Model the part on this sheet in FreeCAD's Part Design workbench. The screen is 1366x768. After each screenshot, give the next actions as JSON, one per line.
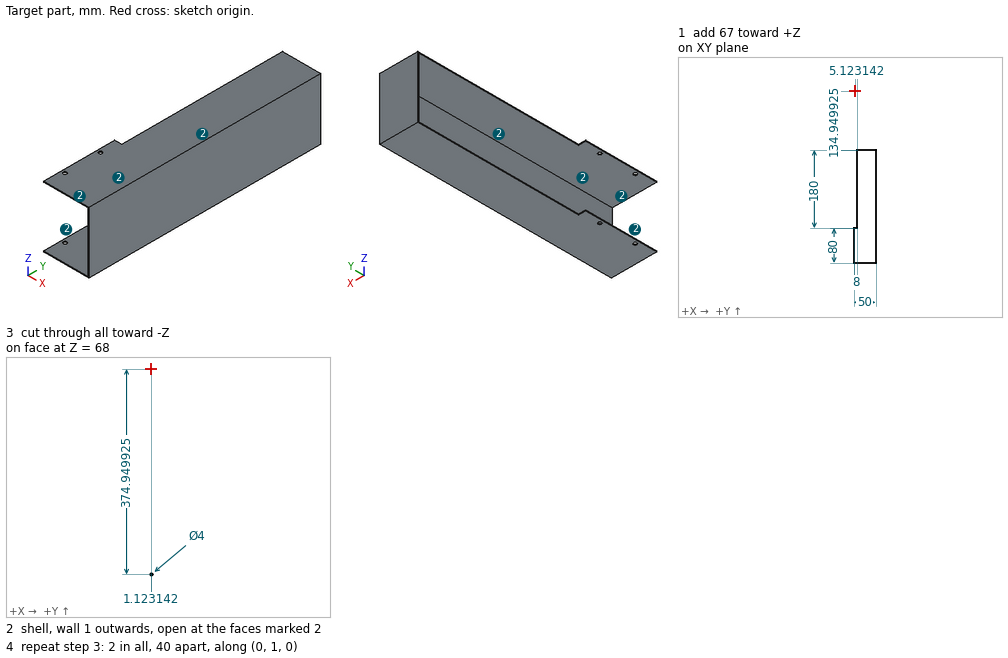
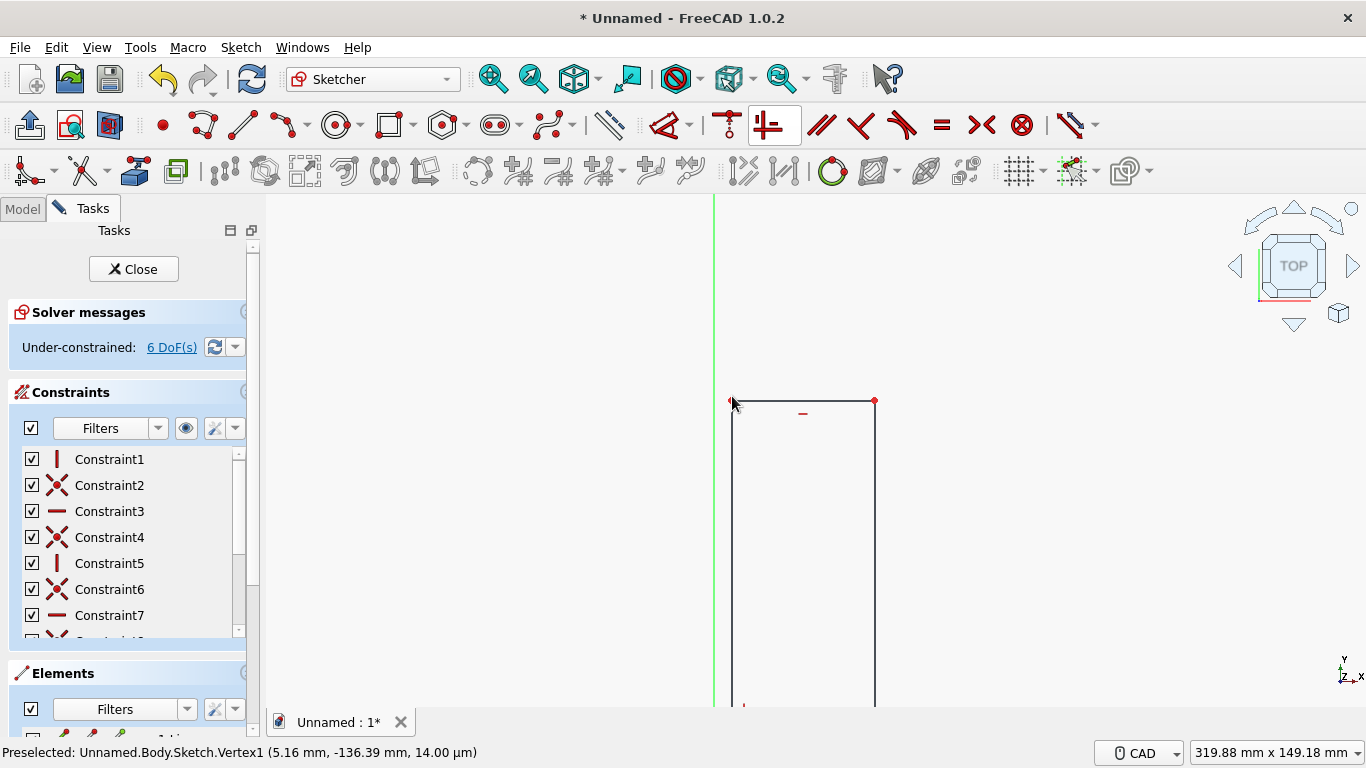
{"action": "left_click", "coordinate": [664, 126]}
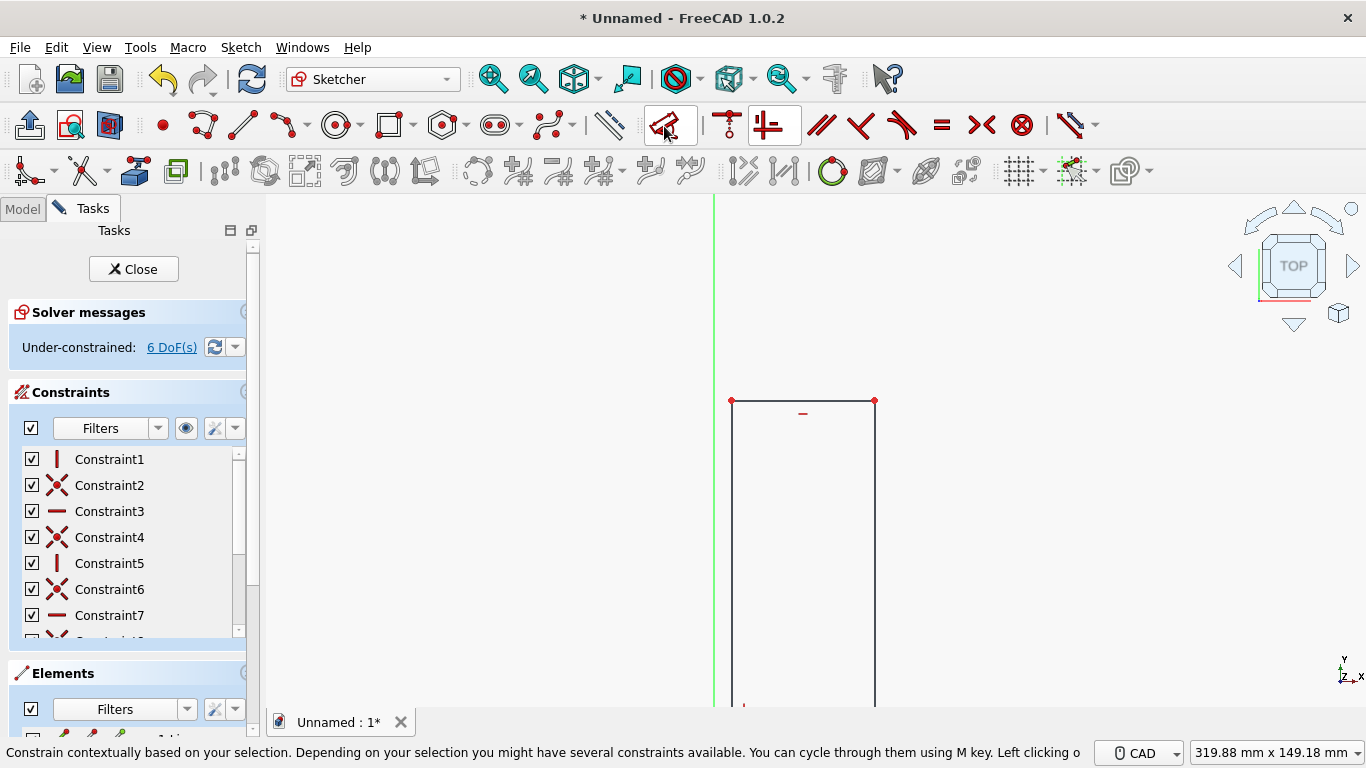
{"action": "scroll", "coordinate": [734, 398], "scroll_direction": "down", "scroll_amount": 7}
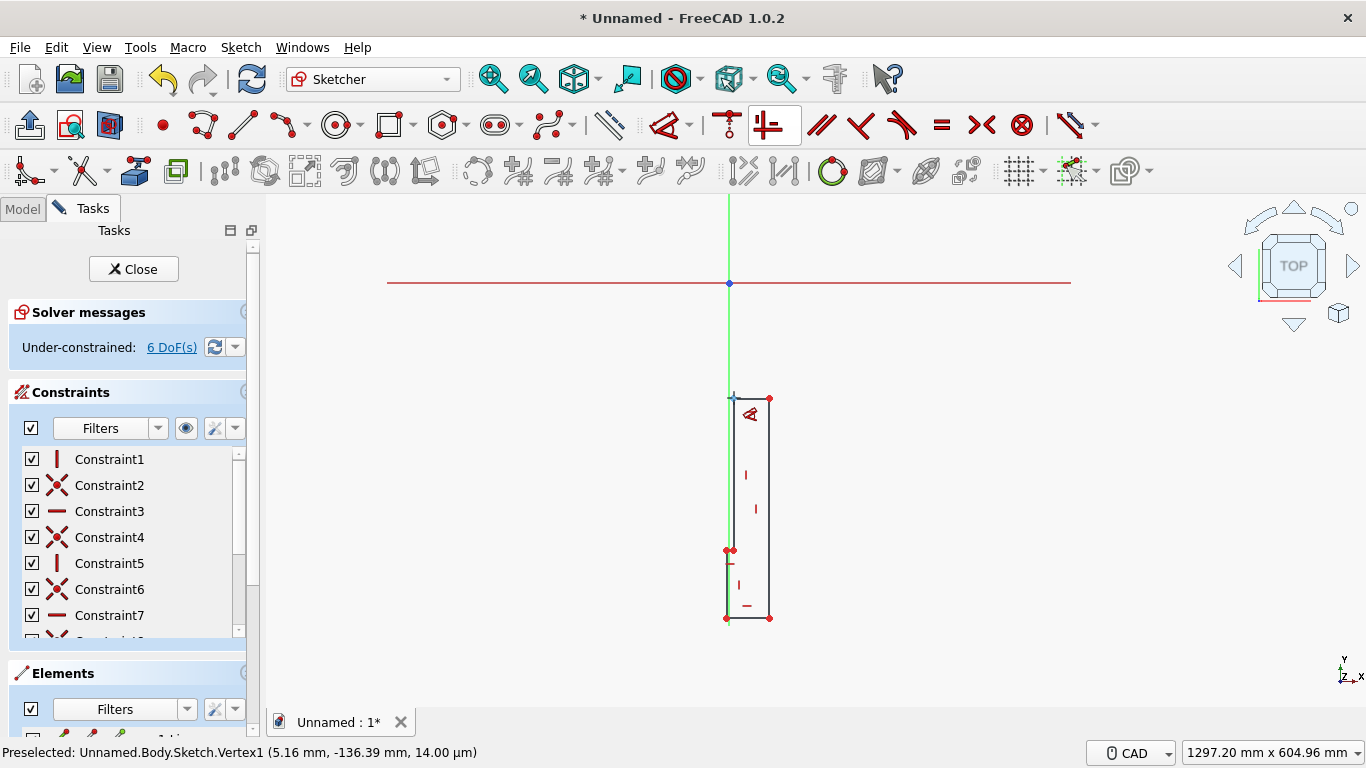
{"action": "scroll", "coordinate": [730, 551], "scroll_direction": "up", "scroll_amount": 9}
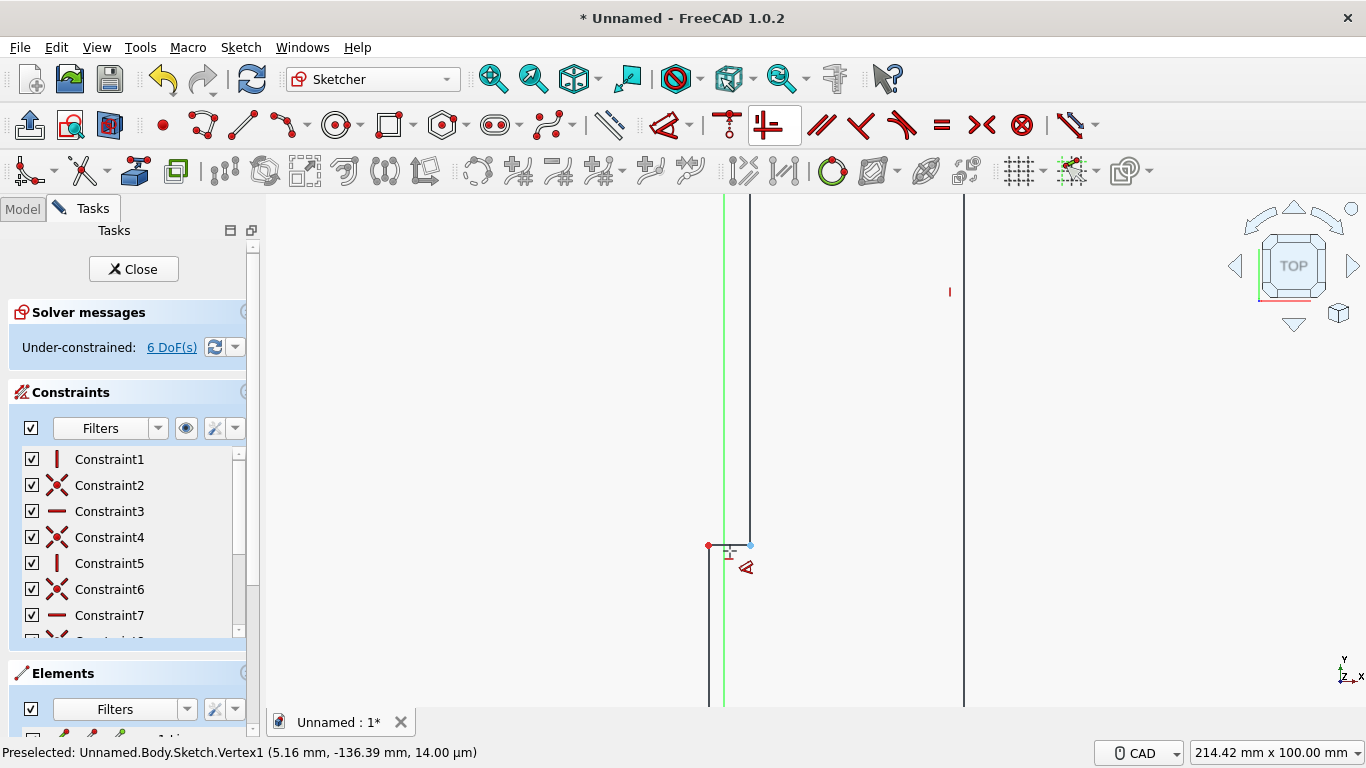
{"action": "left_click", "coordinate": [725, 545]}
{"action": "left_click", "coordinate": [739, 579]}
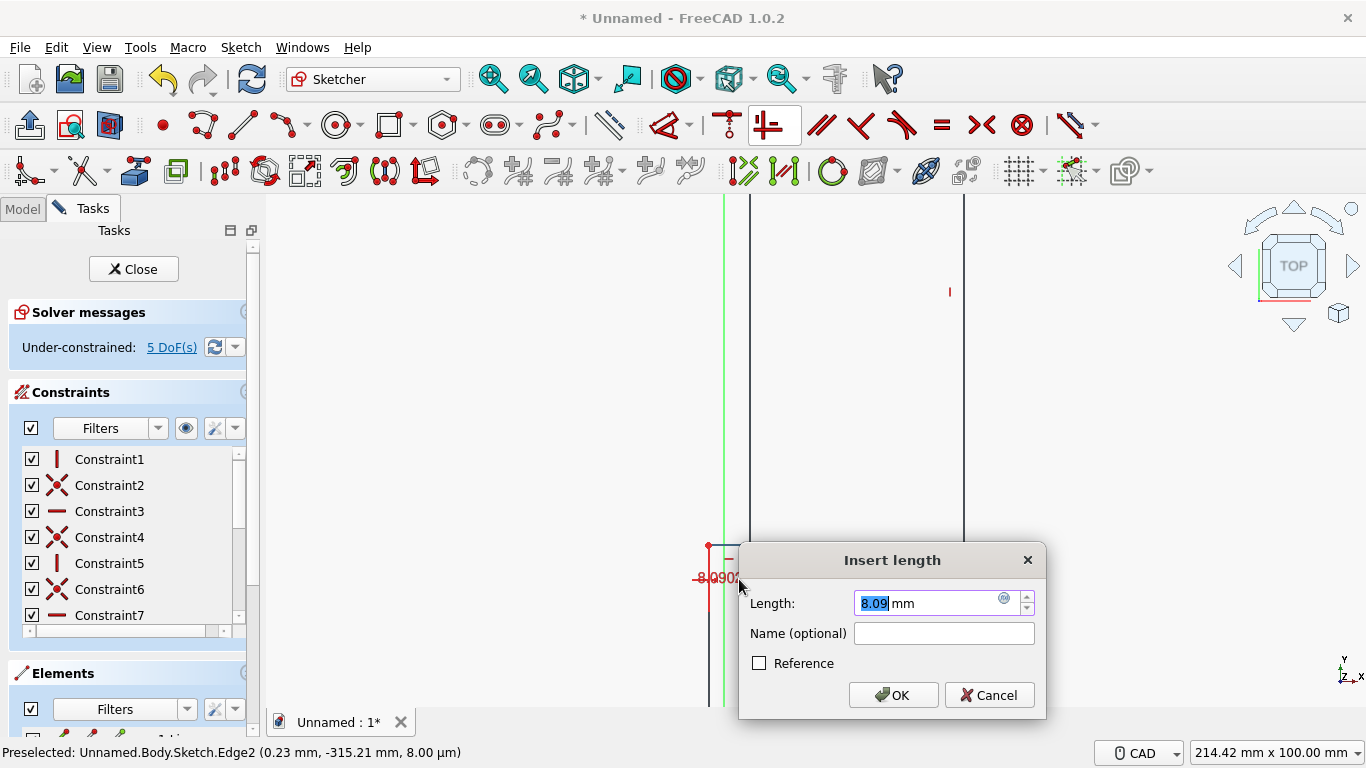
{"action": "type", "text": "8"}
{"action": "key", "text": "Return"}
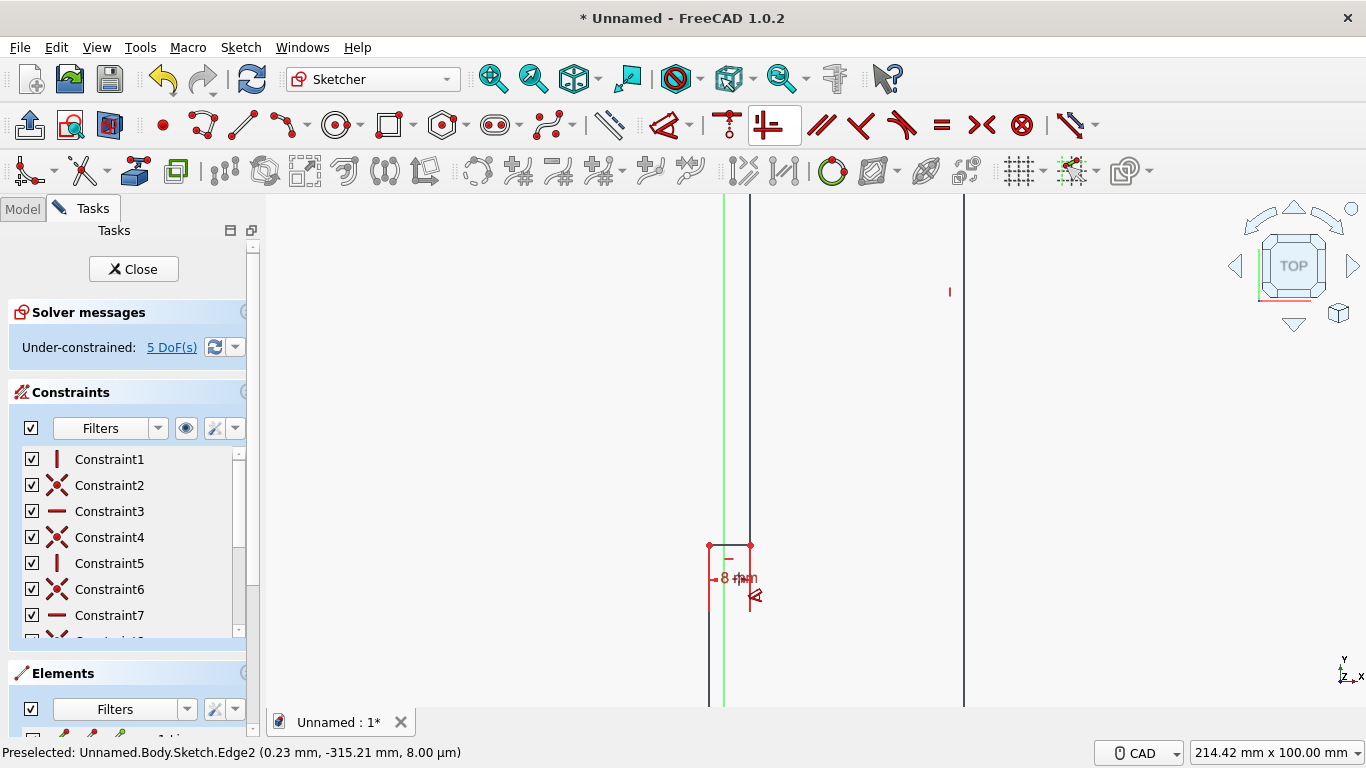
{"action": "left_click", "coordinate": [709, 668]}
{"action": "left_click", "coordinate": [675, 612]}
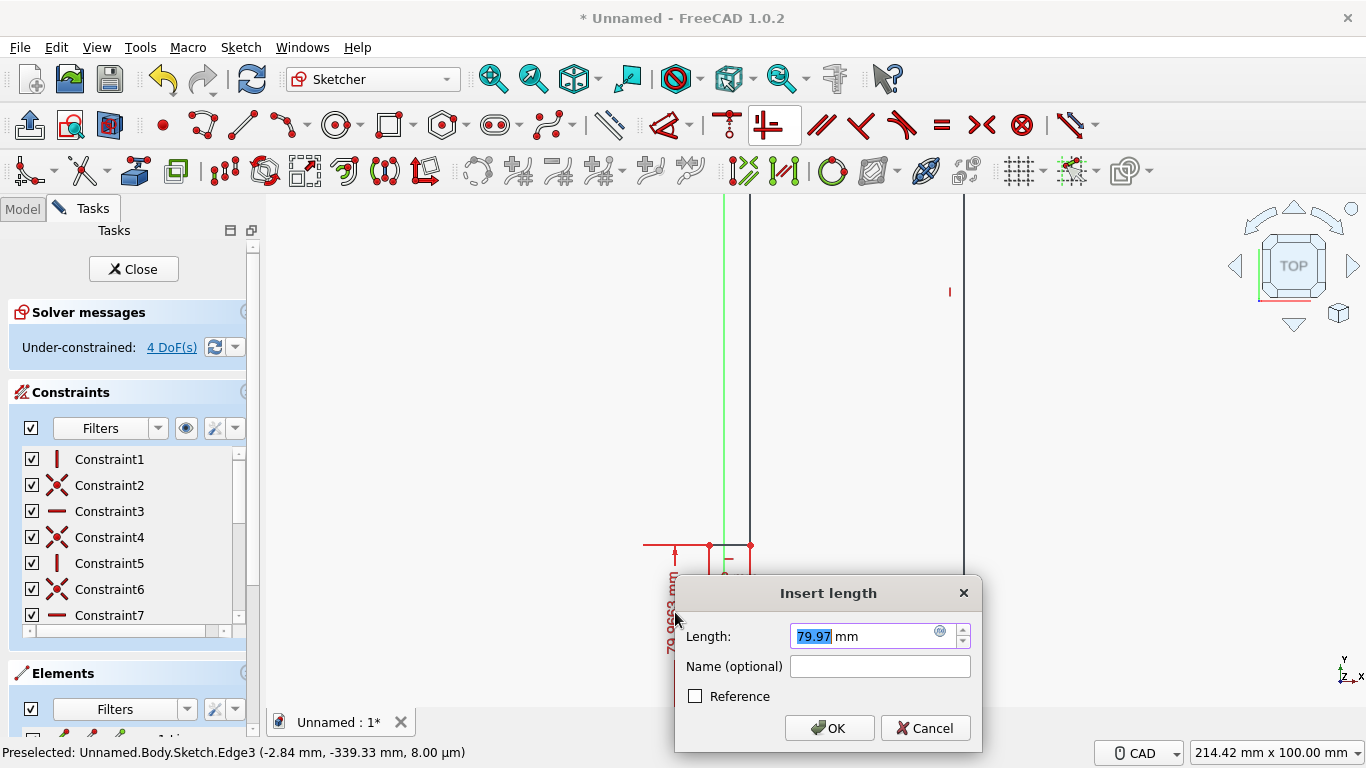
{"action": "type", "text": "80"}
{"action": "key", "text": "Return"}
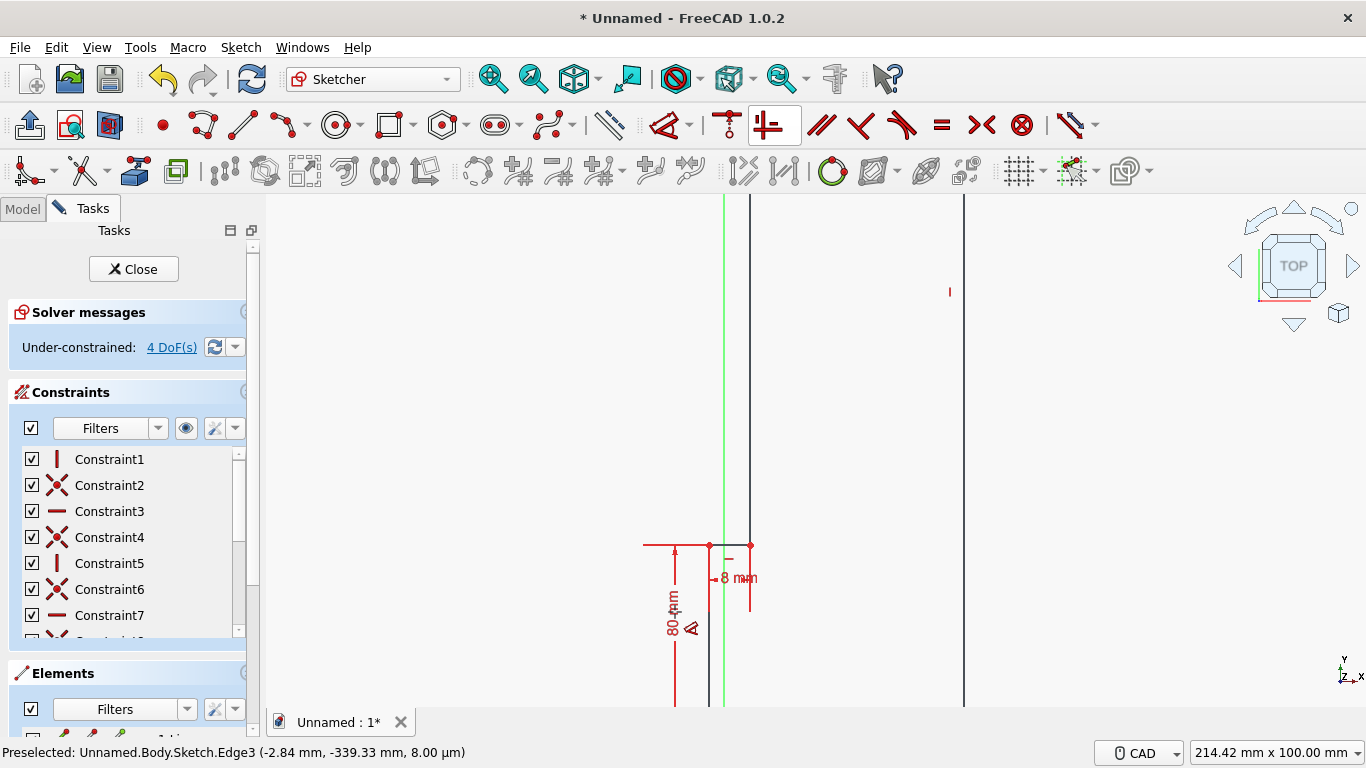
{"action": "scroll", "coordinate": [730, 551], "scroll_direction": "down", "scroll_amount": 9}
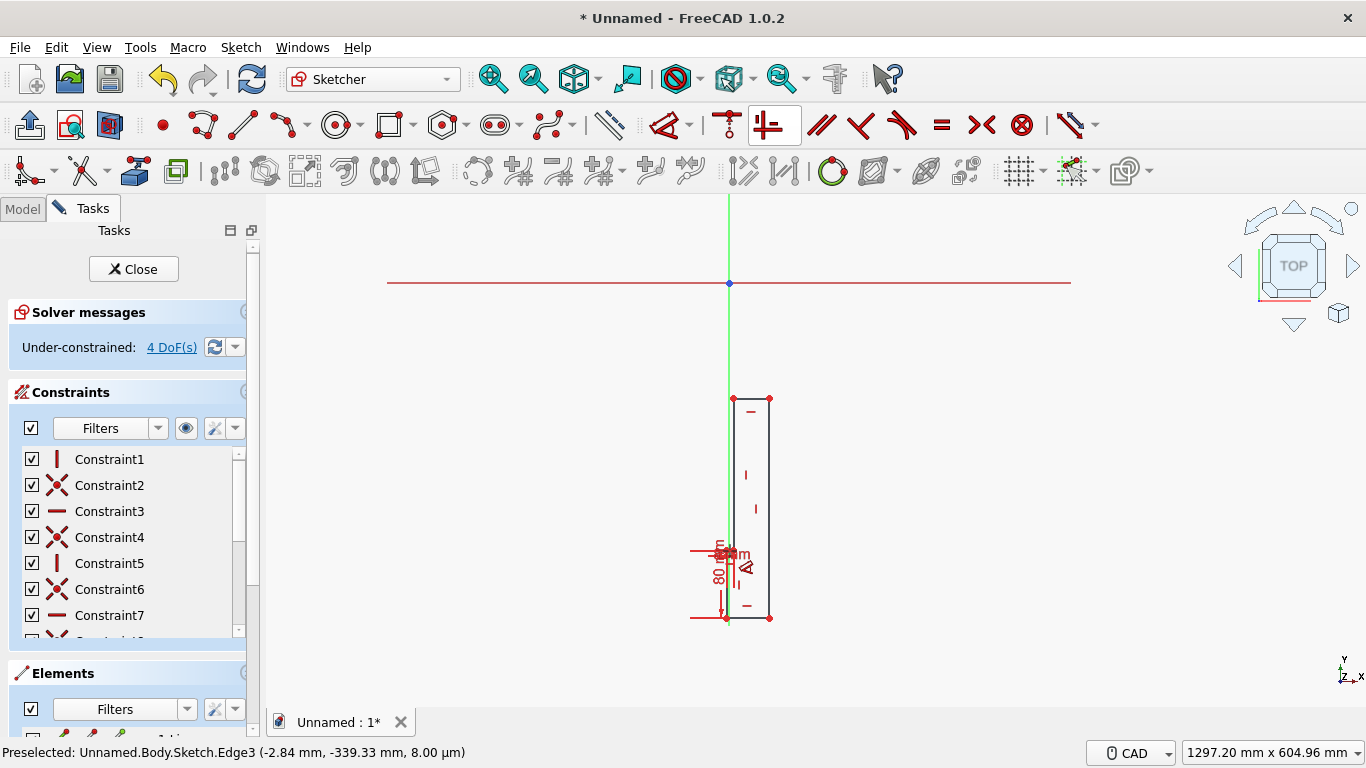
{"action": "scroll", "coordinate": [740, 618], "scroll_direction": "up", "scroll_amount": 2}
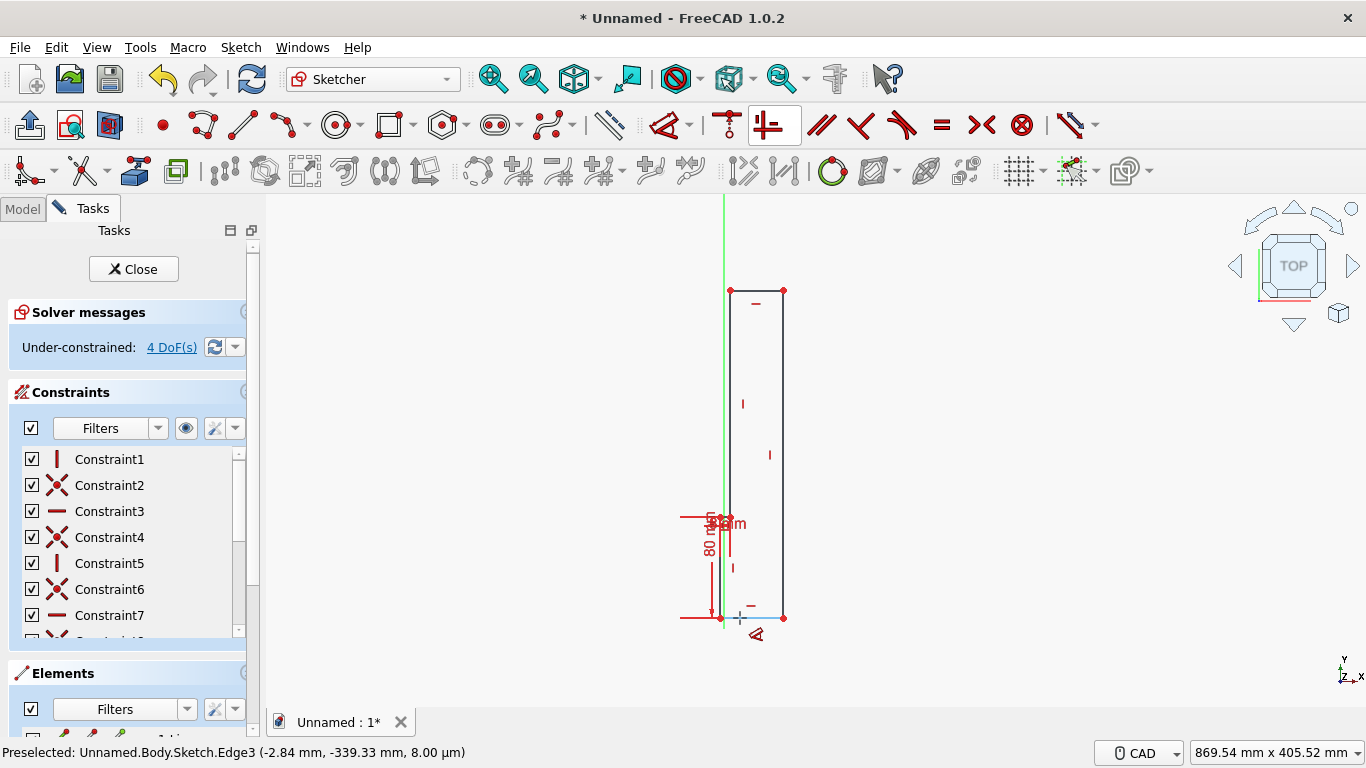
{"action": "left_click", "coordinate": [739, 618]}
{"action": "left_click", "coordinate": [752, 652]}